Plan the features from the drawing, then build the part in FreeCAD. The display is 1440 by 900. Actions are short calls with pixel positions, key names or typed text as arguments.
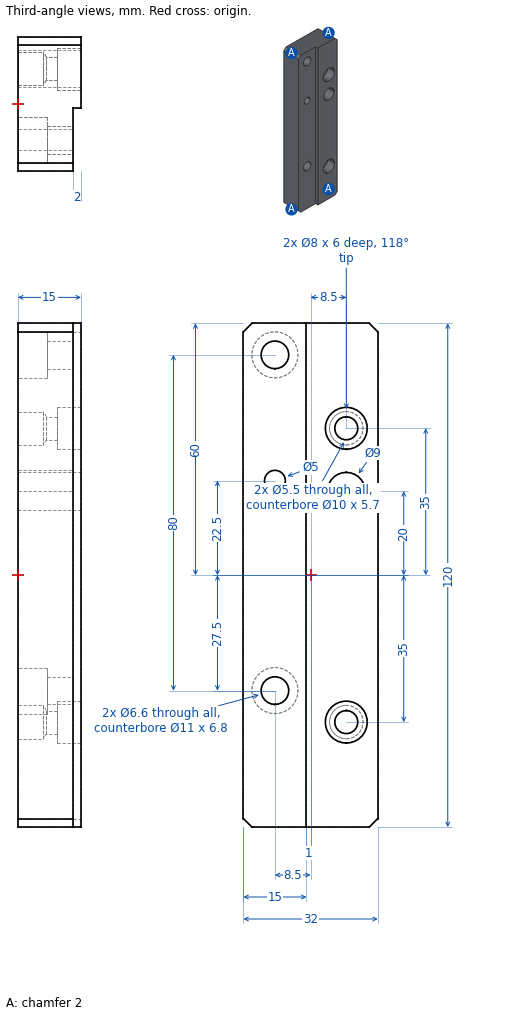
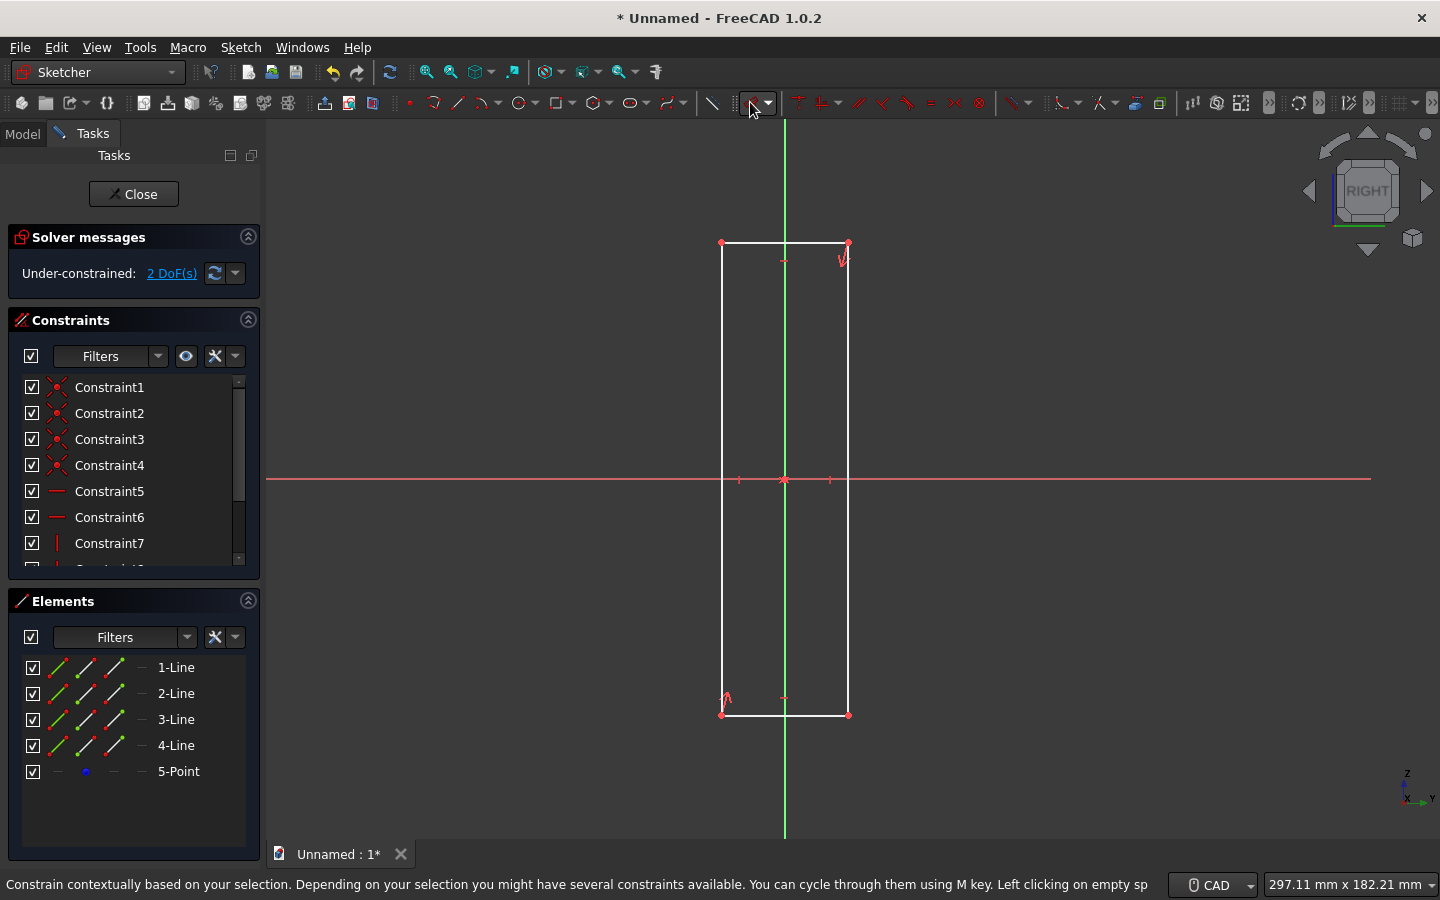
click(759, 716)
click(756, 750)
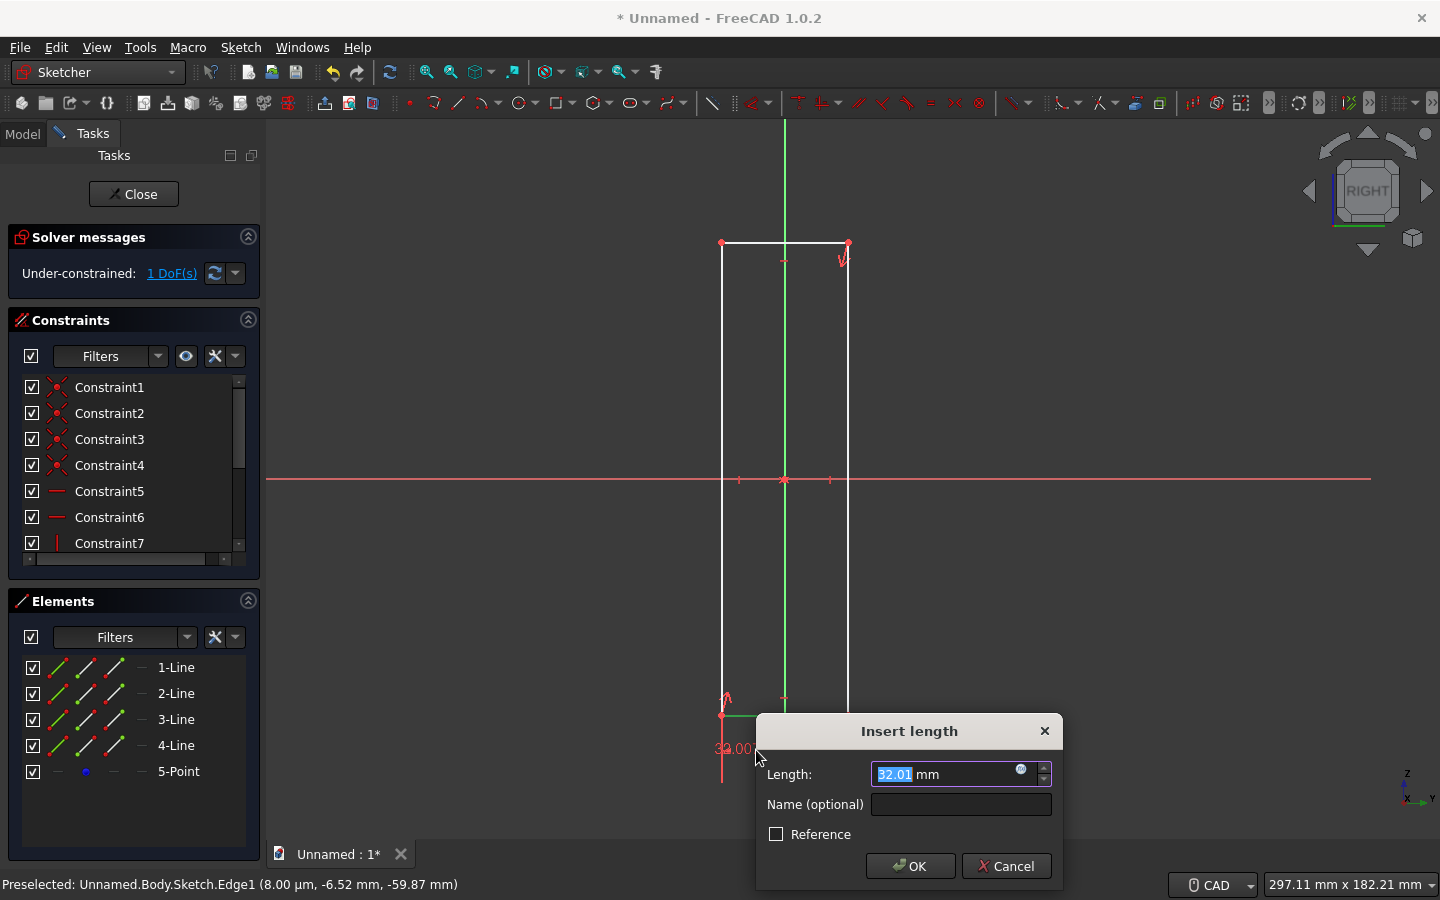
text(32)
key(Return)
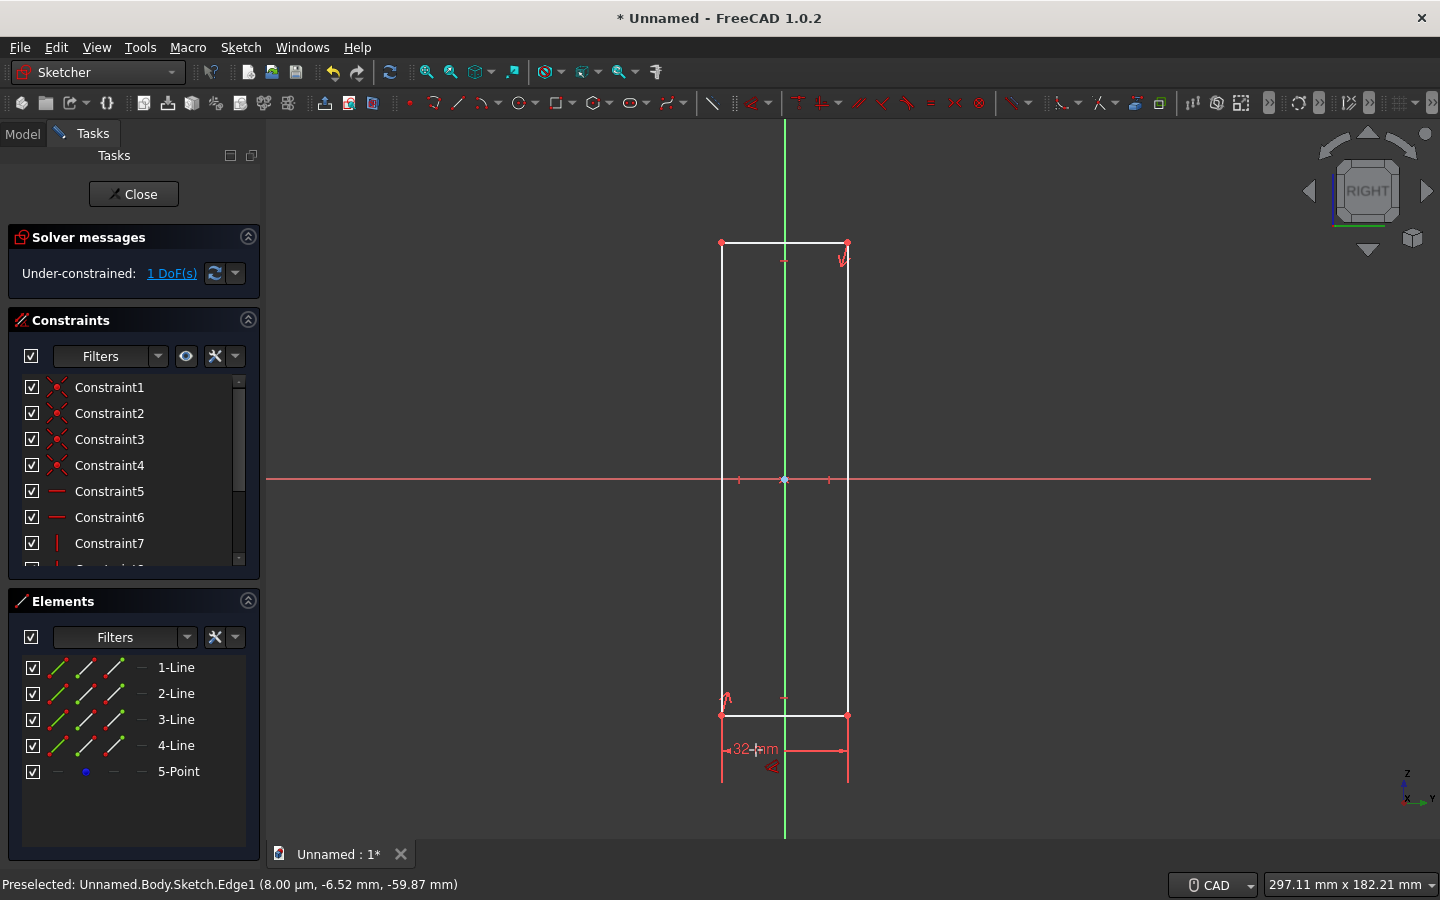
click(848, 574)
click(882, 370)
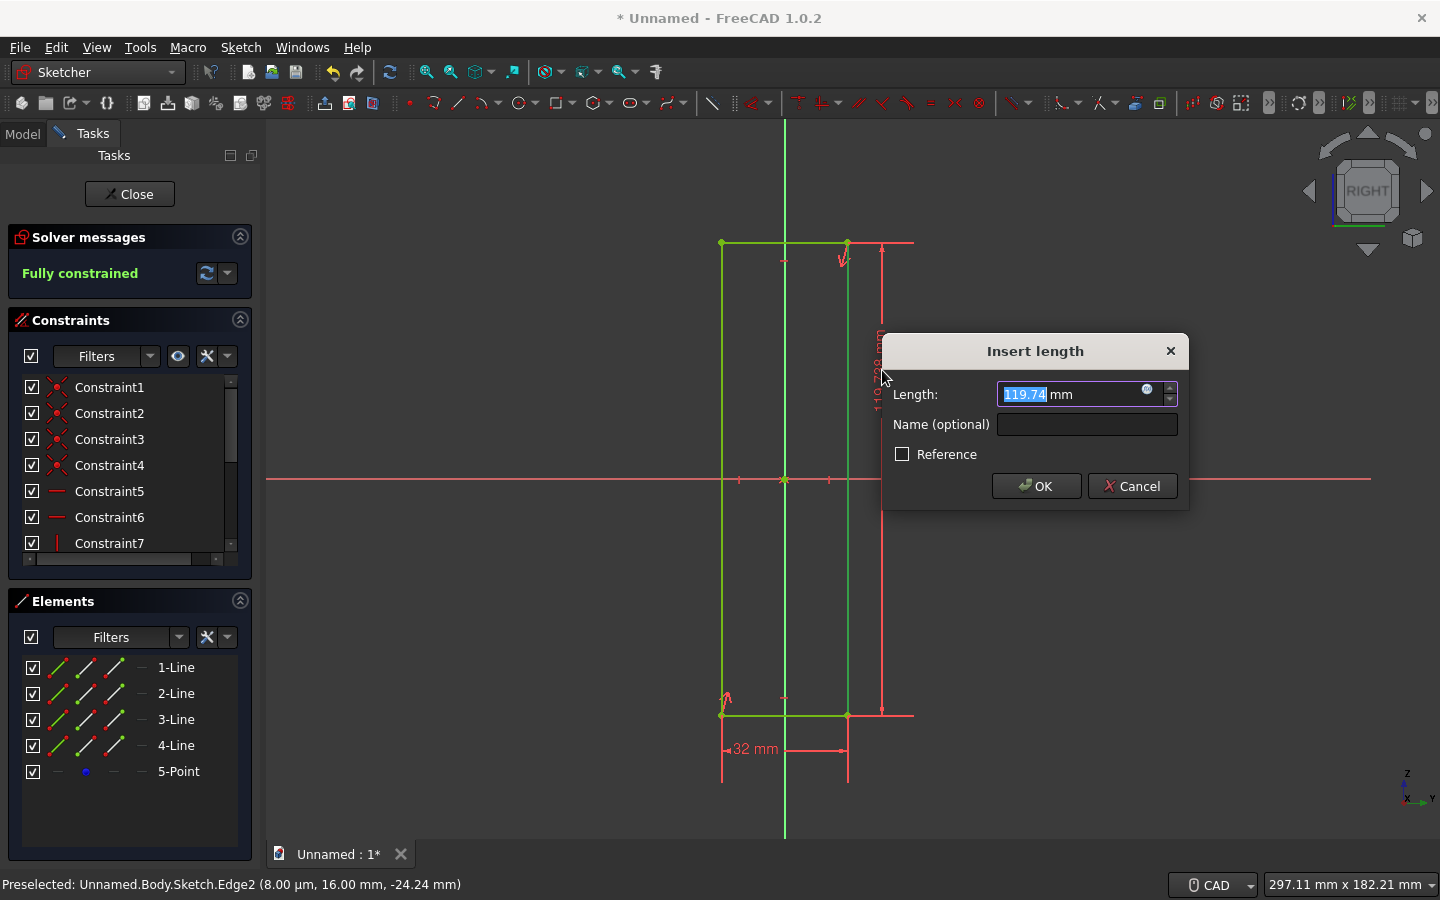
text(120)
key(Return)
key(Escape)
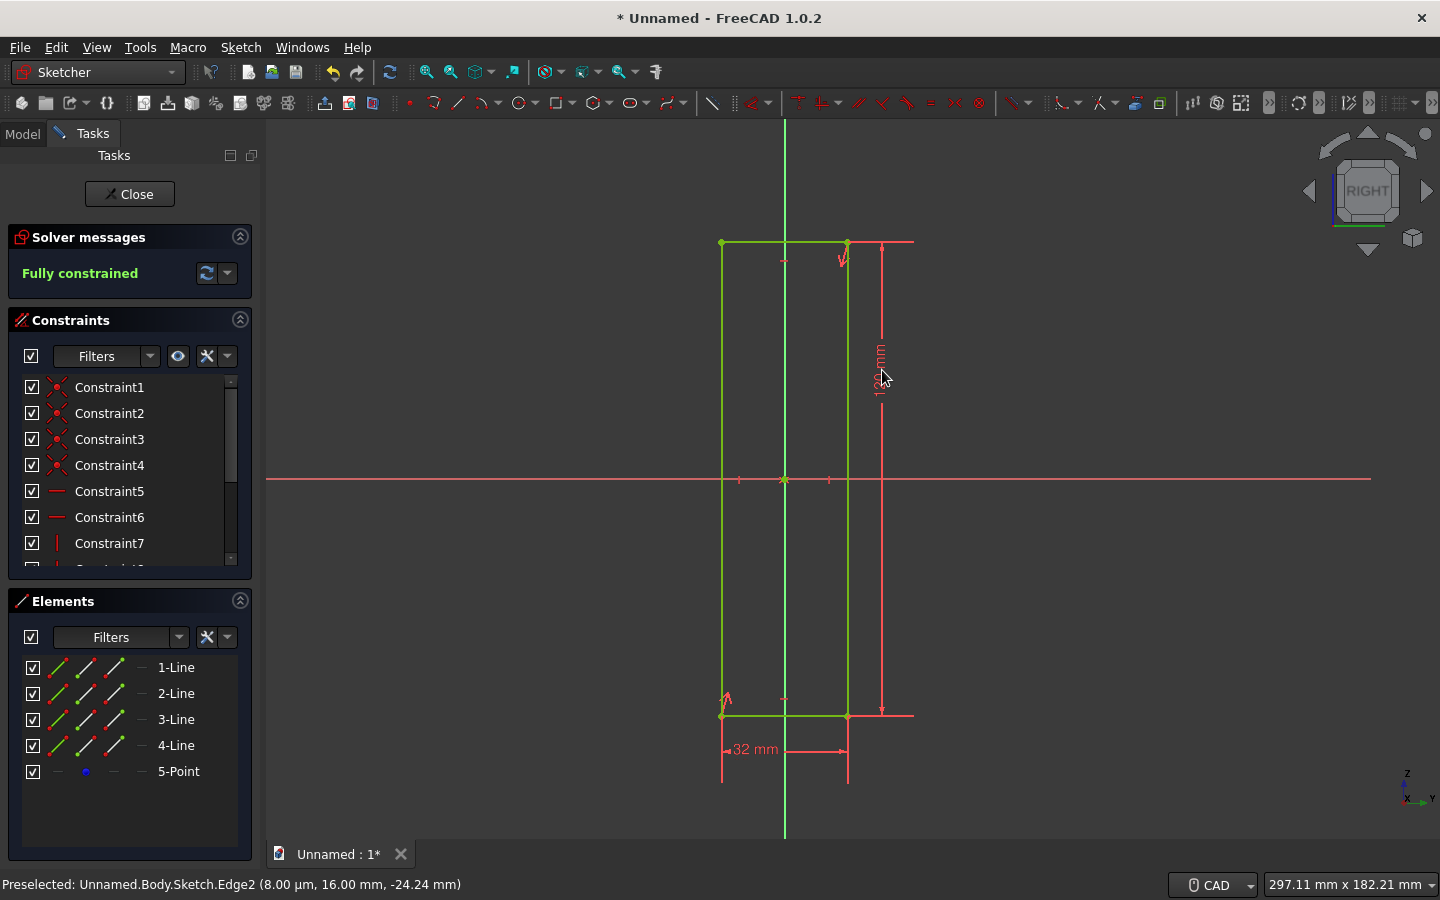
click(130, 194)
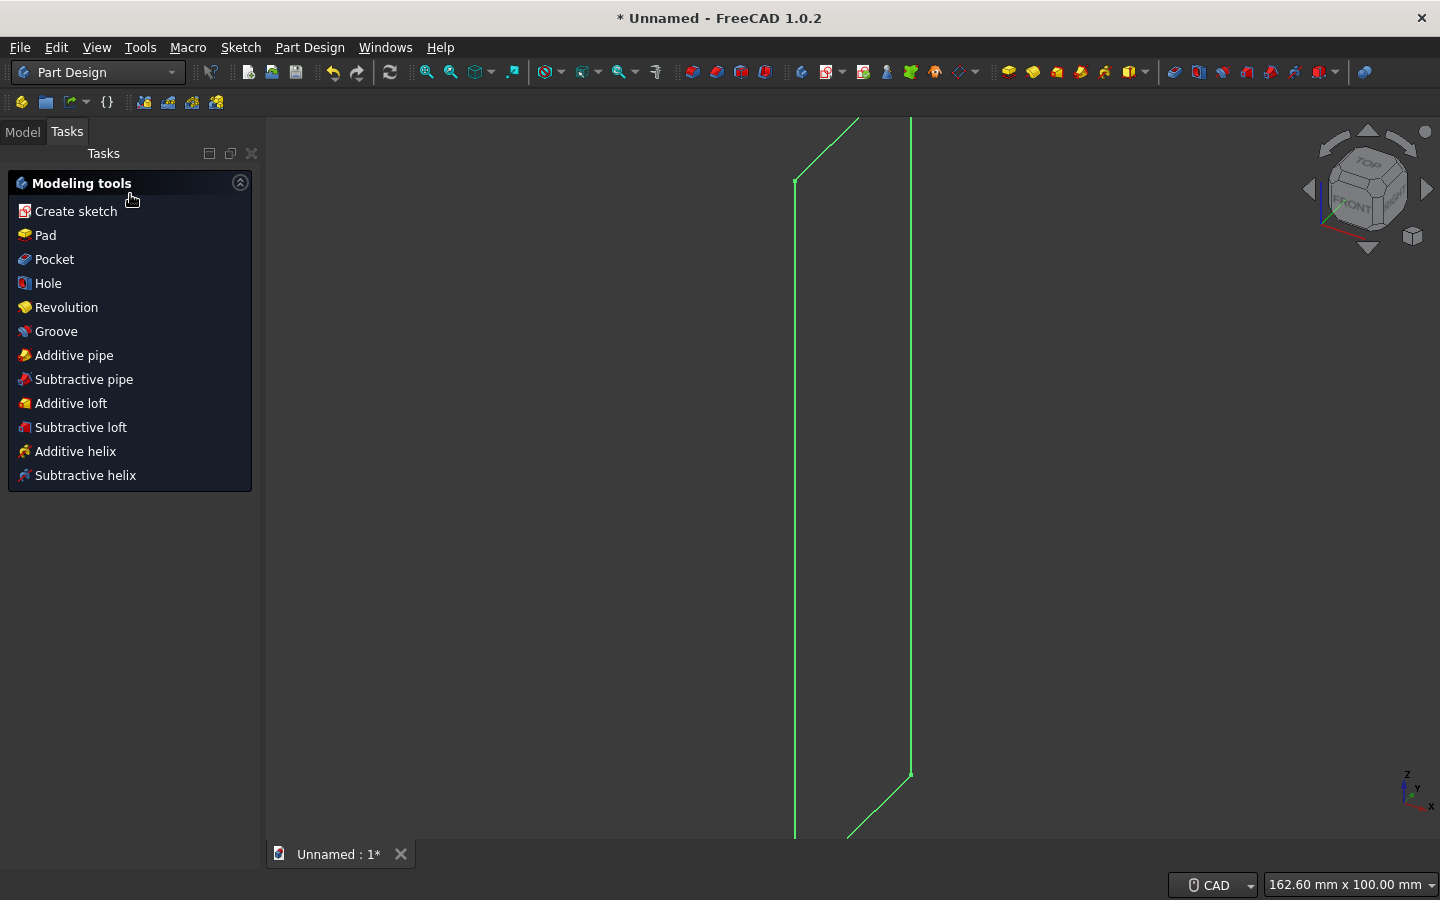
click(1010, 72)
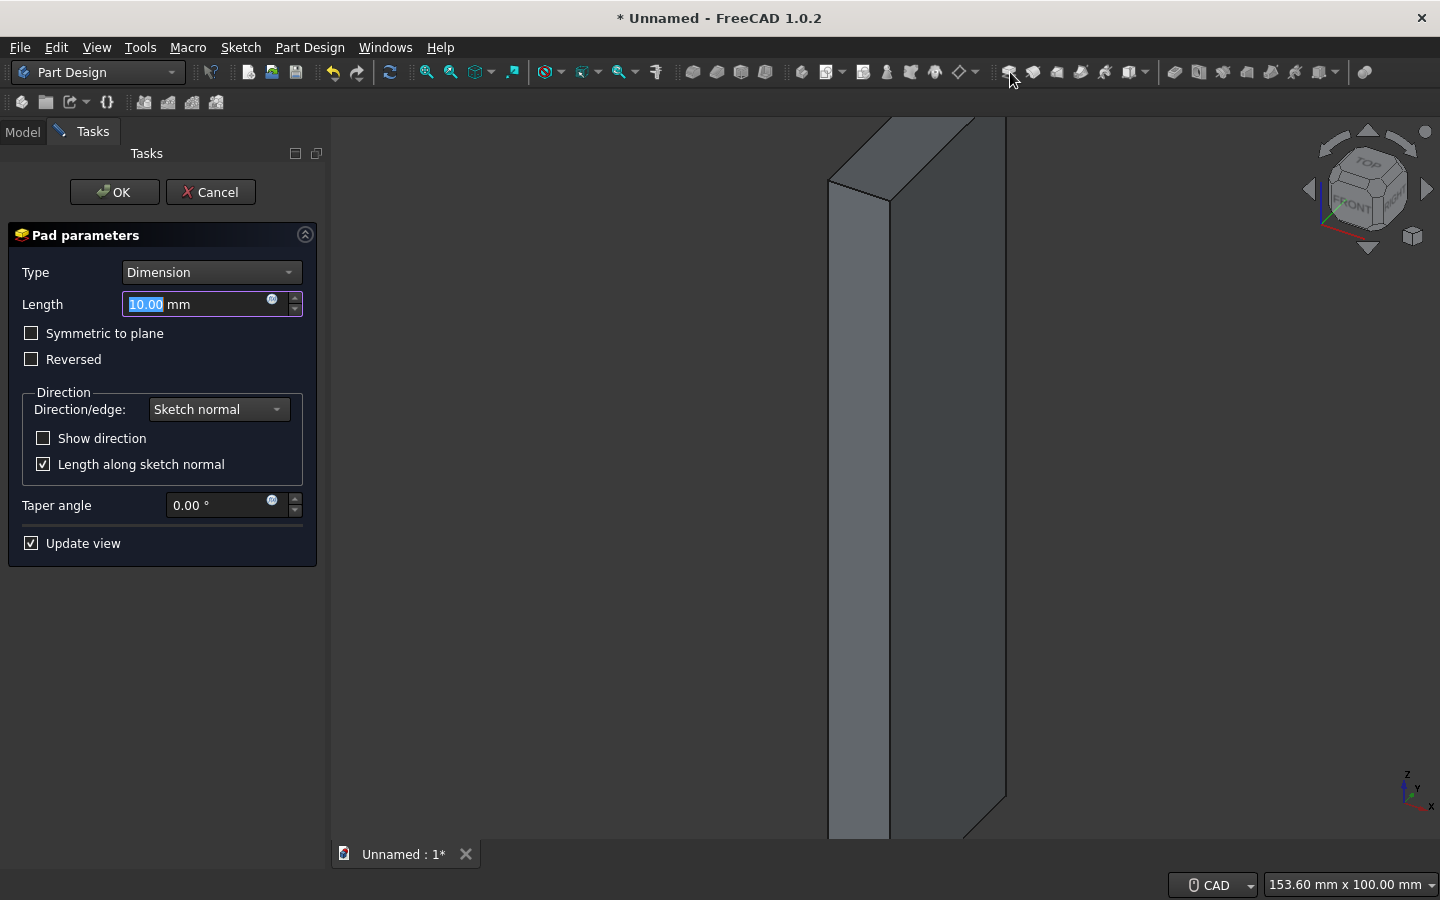
text(15)
key(Tab)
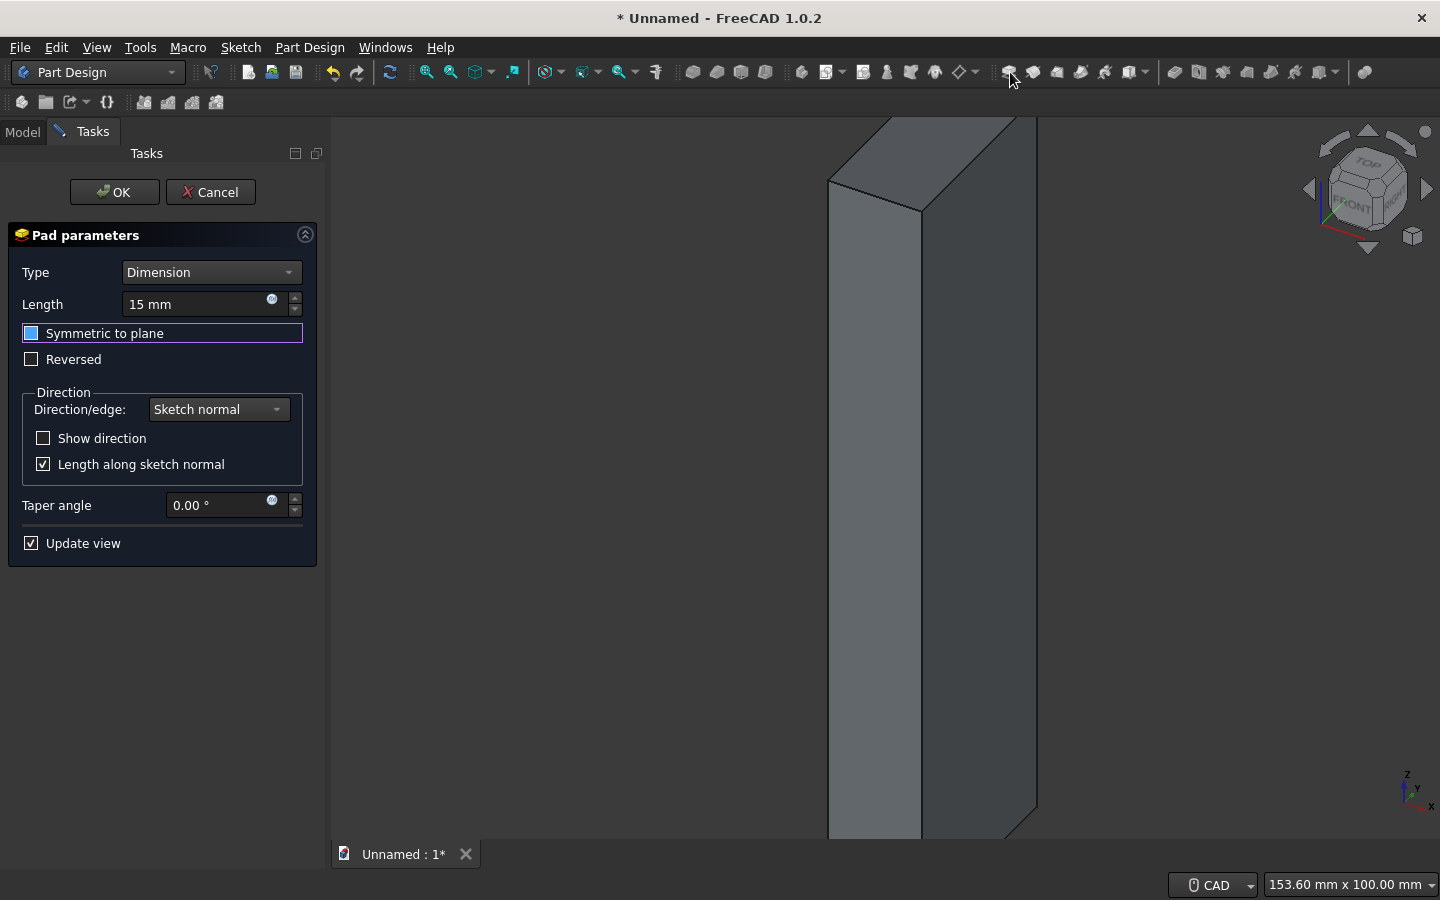
click(115, 192)